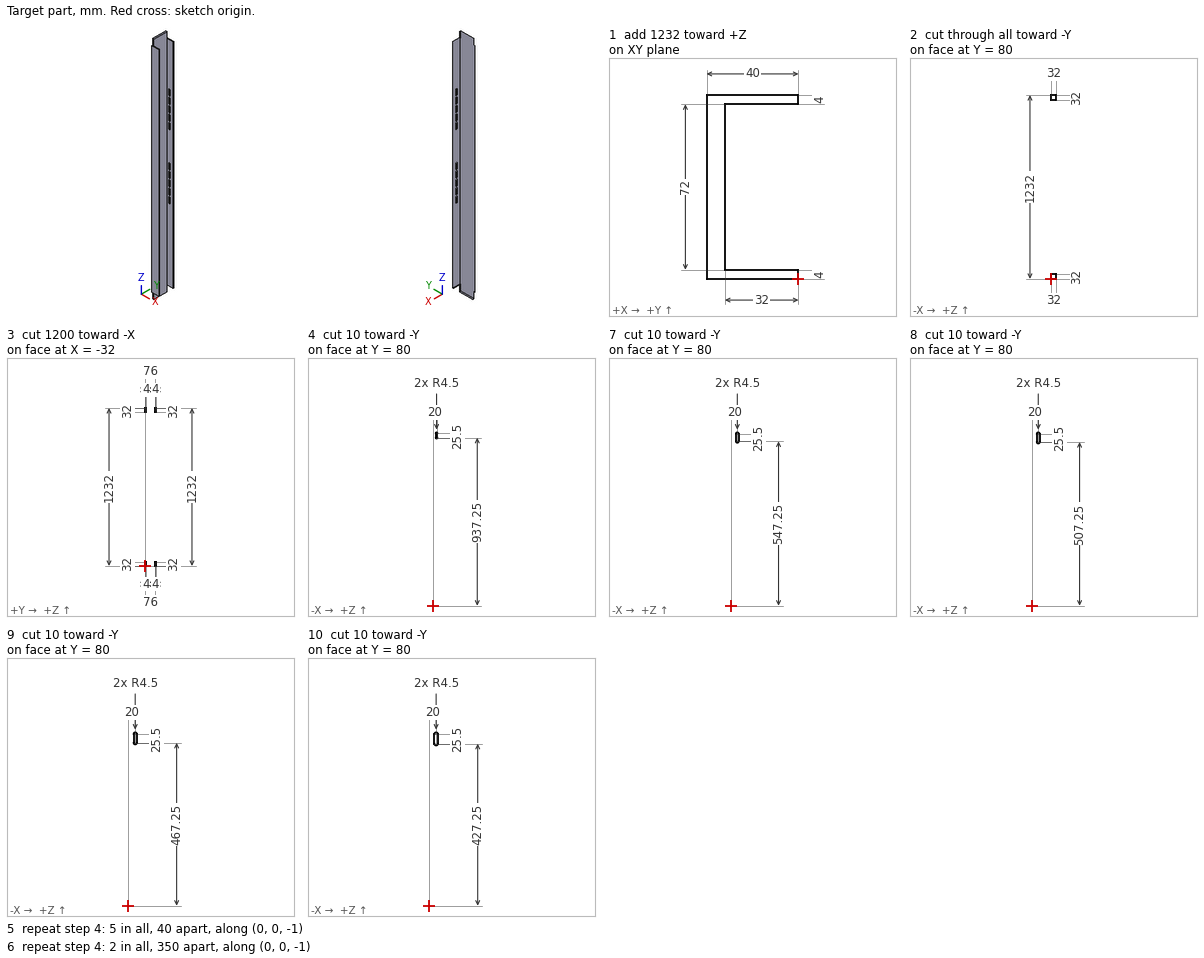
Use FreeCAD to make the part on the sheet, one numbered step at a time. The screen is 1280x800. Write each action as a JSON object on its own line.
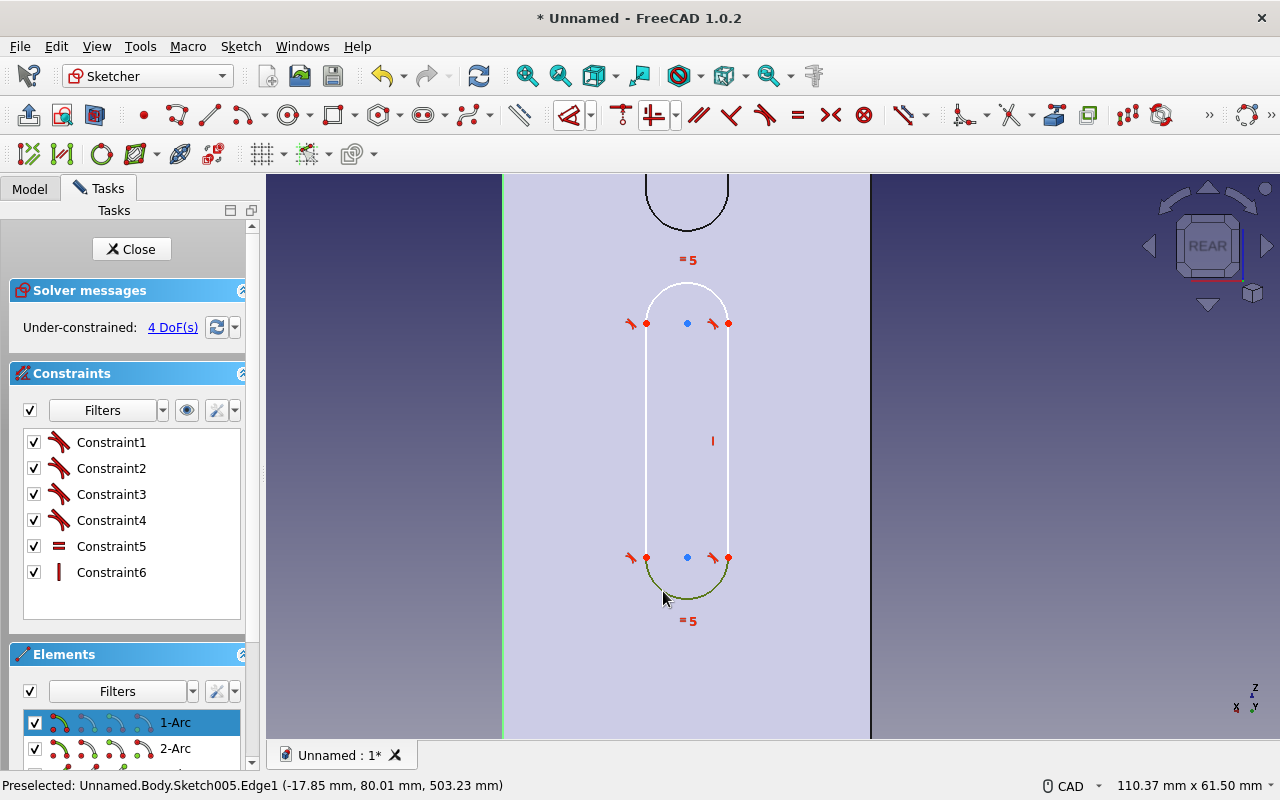
{"action": "key", "text": "k r"}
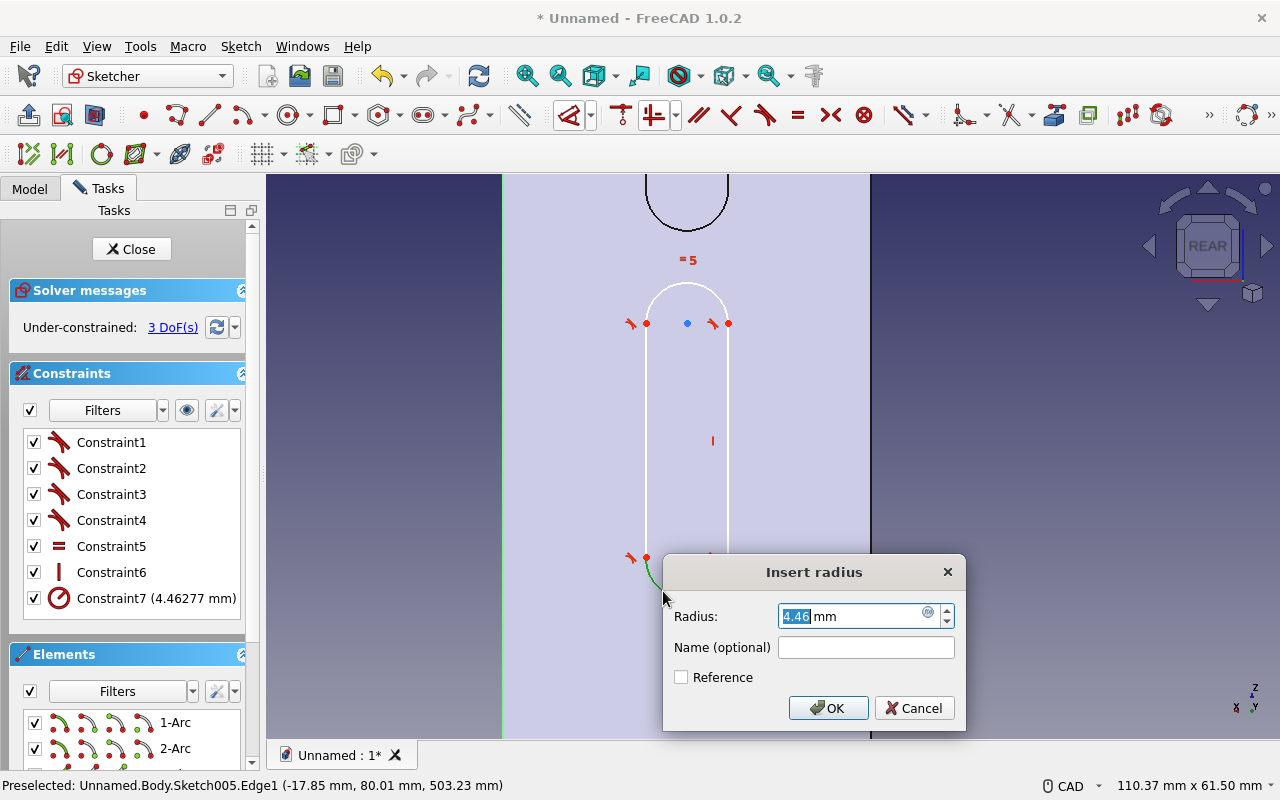
{"action": "type", "text": "4.5"}
{"action": "key", "text": "Return"}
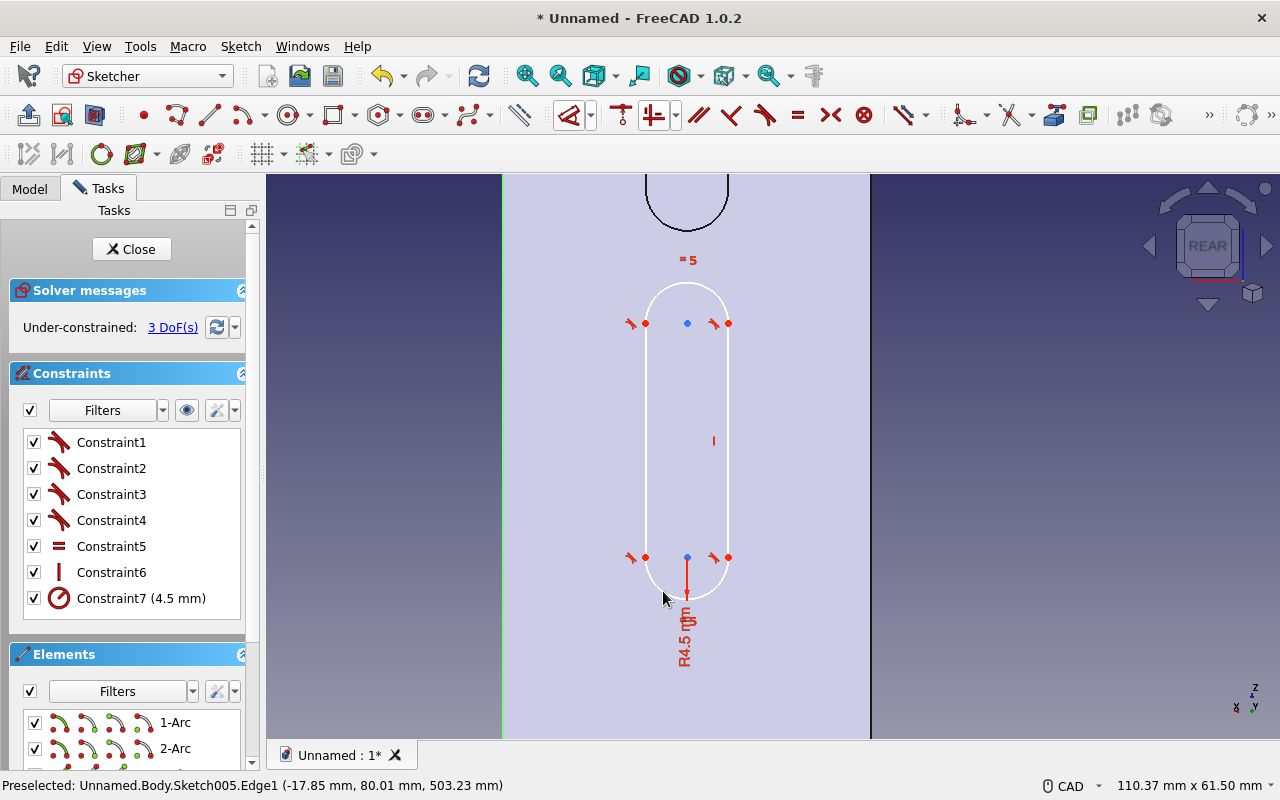
{"action": "left_click", "coordinate": [687, 558]}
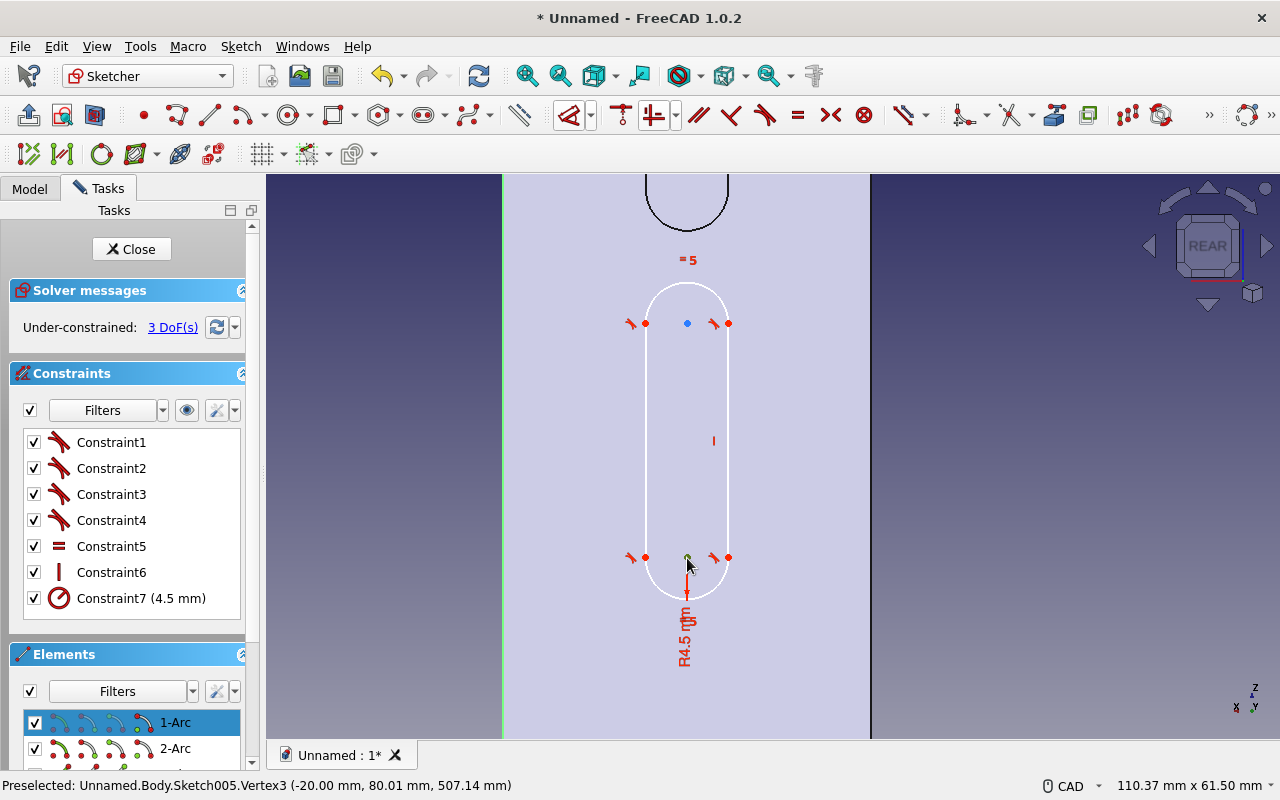
{"action": "left_click", "coordinate": [590, 116]}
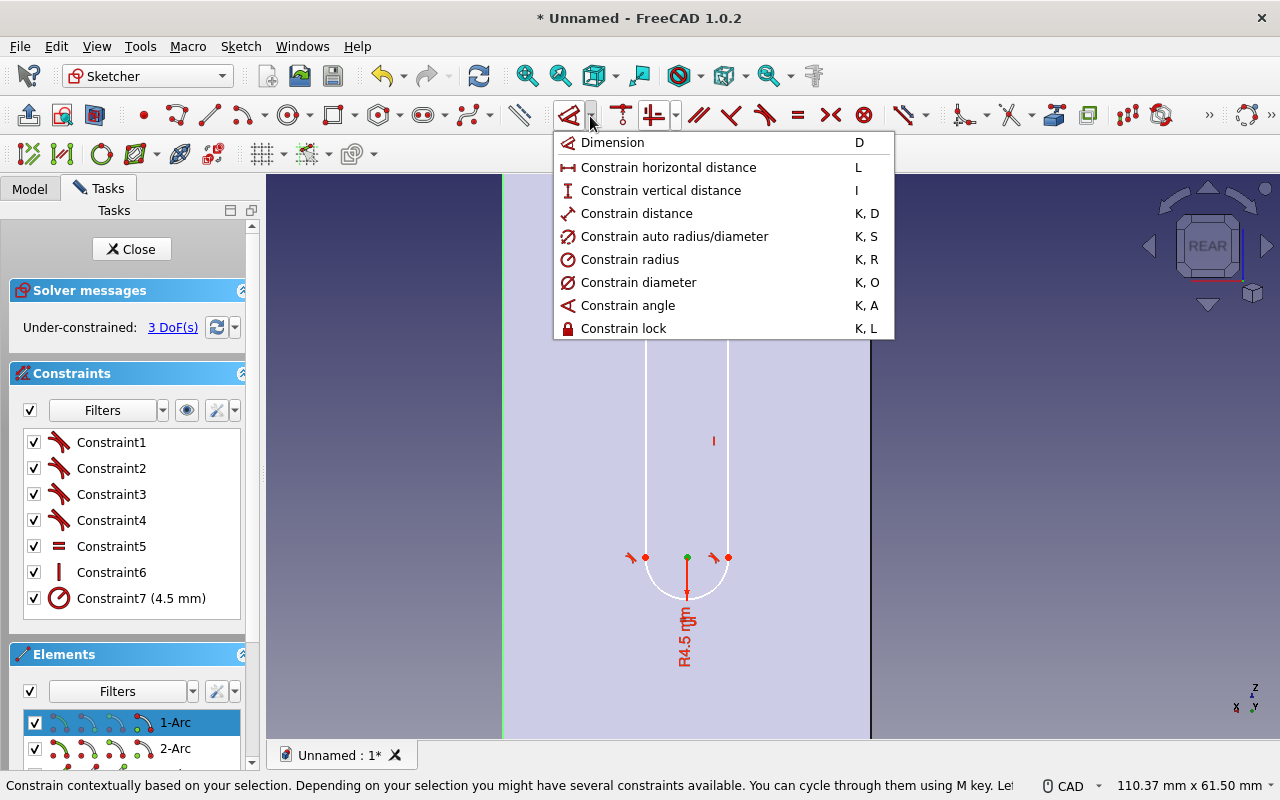
{"action": "left_click", "coordinate": [724, 168]}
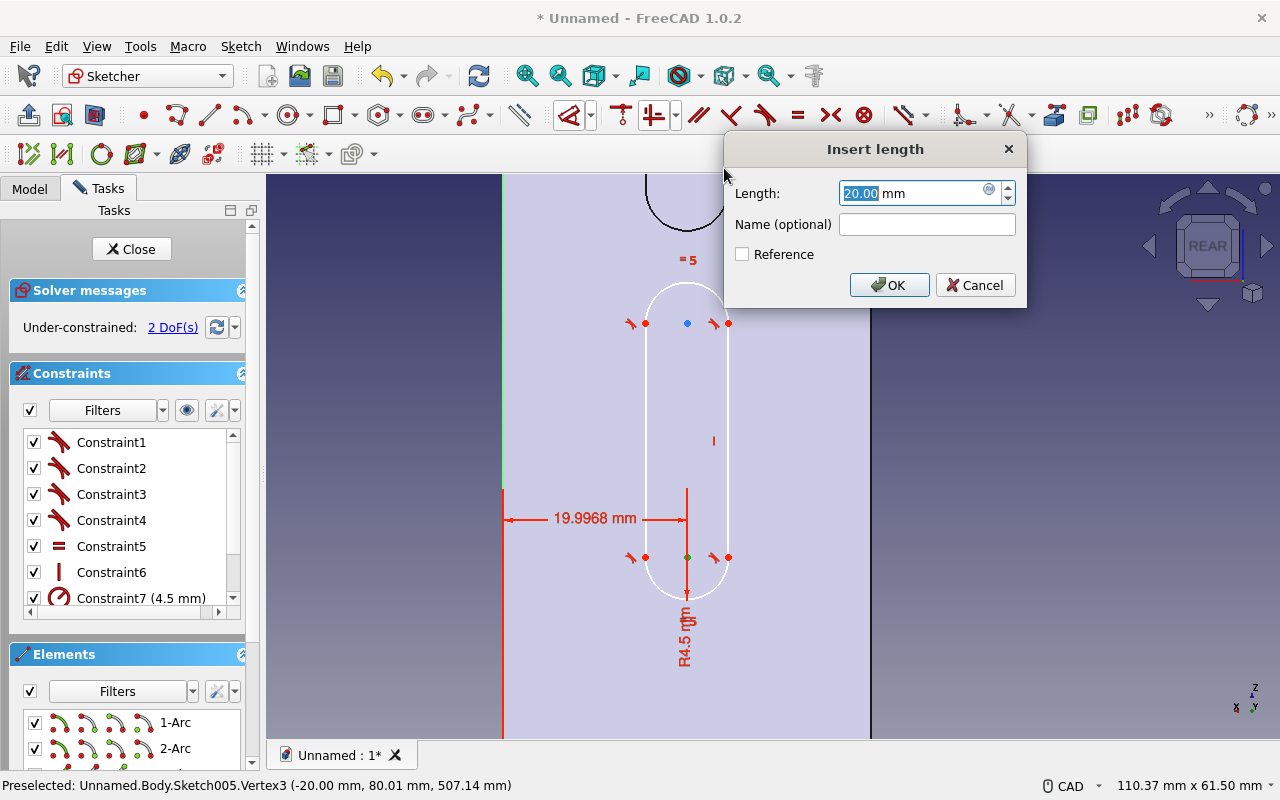
{"action": "type", "text": "20"}
{"action": "key", "text": "Return"}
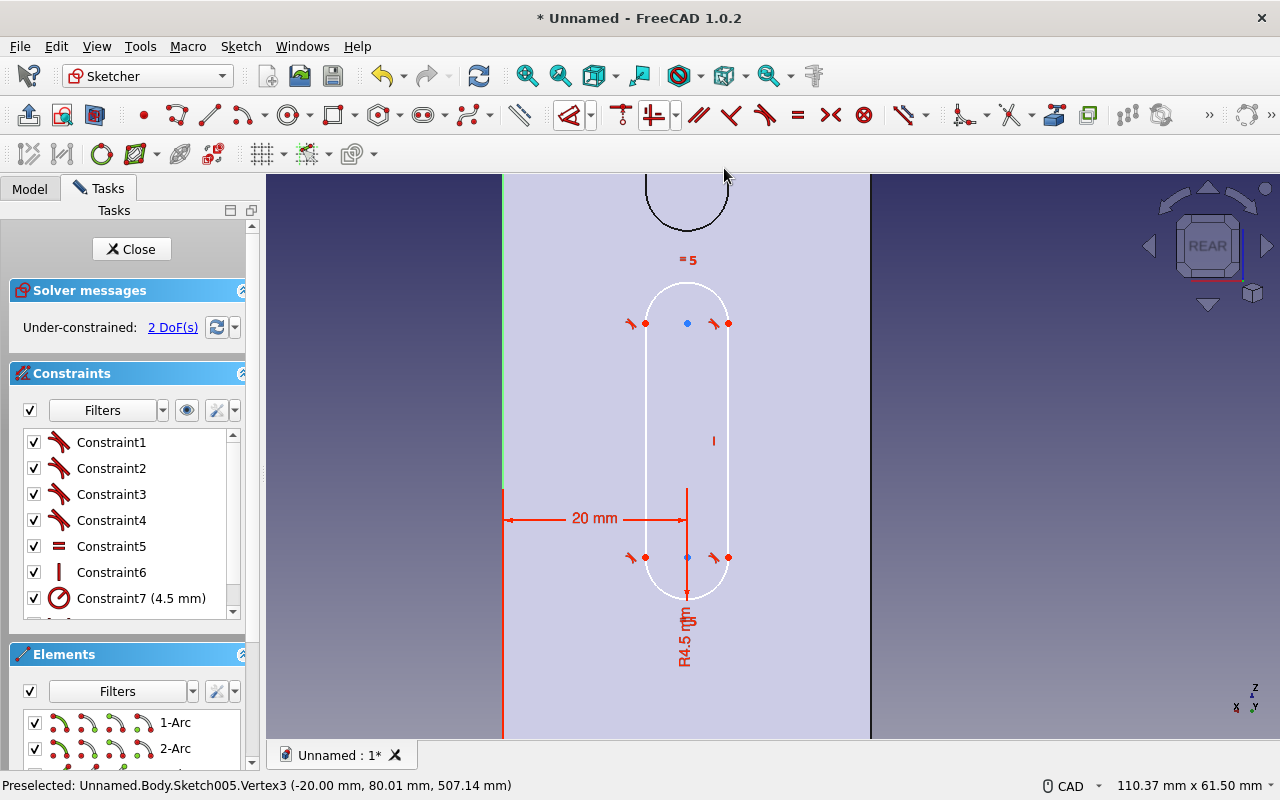
{"action": "left_click", "coordinate": [646, 488]}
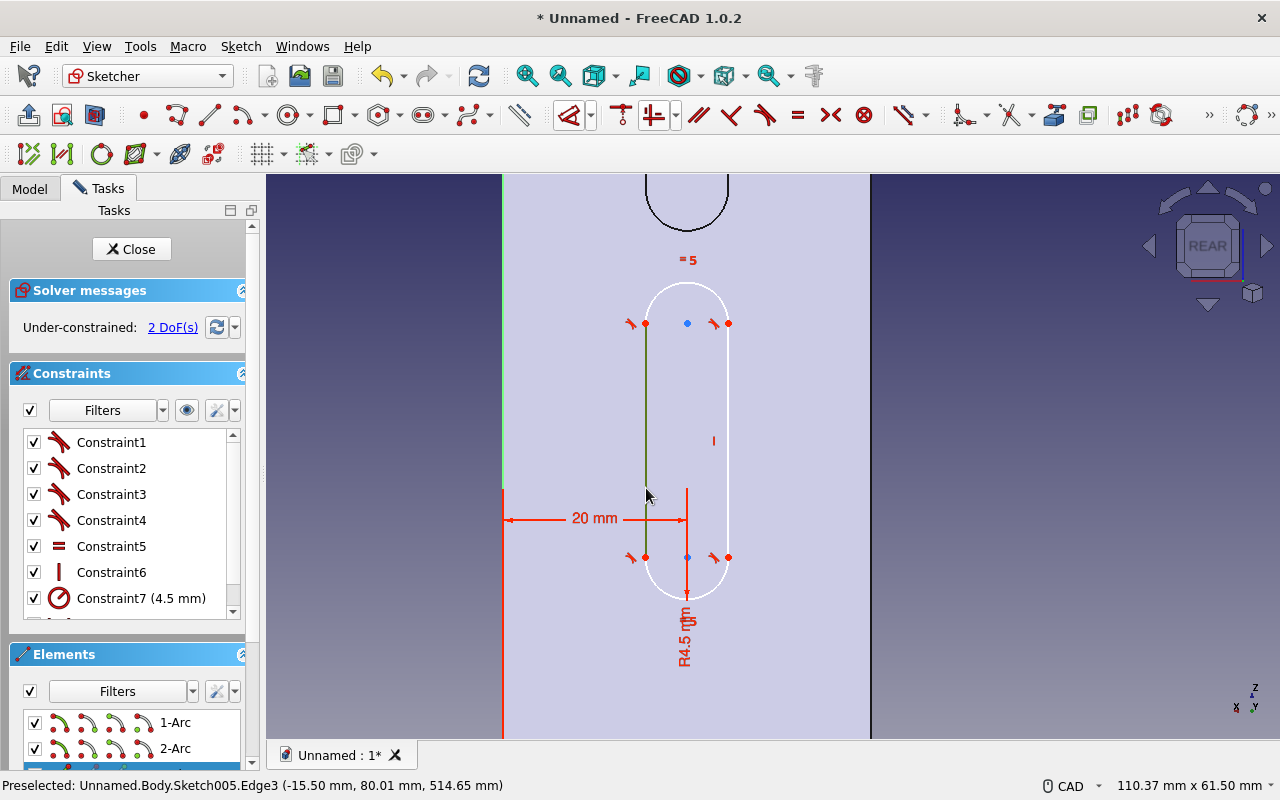
{"action": "left_click", "coordinate": [590, 116]}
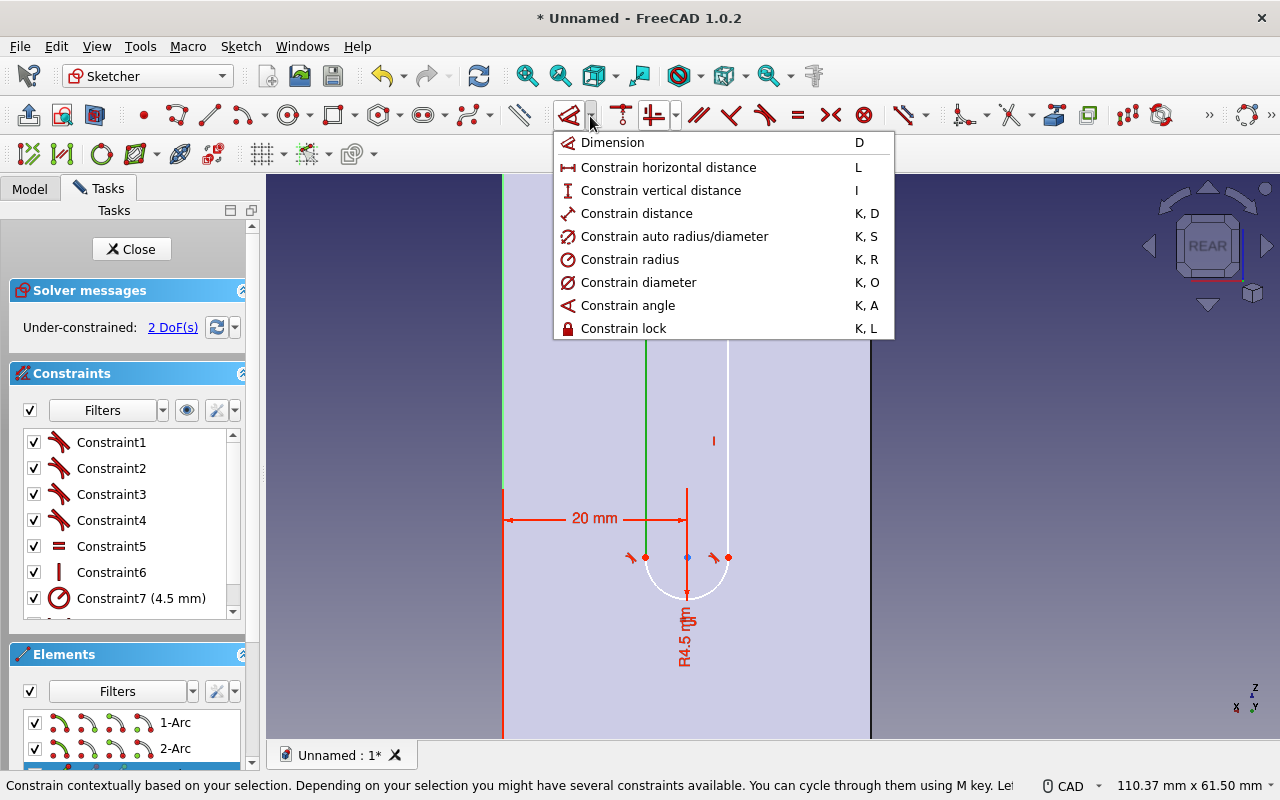
{"action": "left_click", "coordinate": [724, 190]}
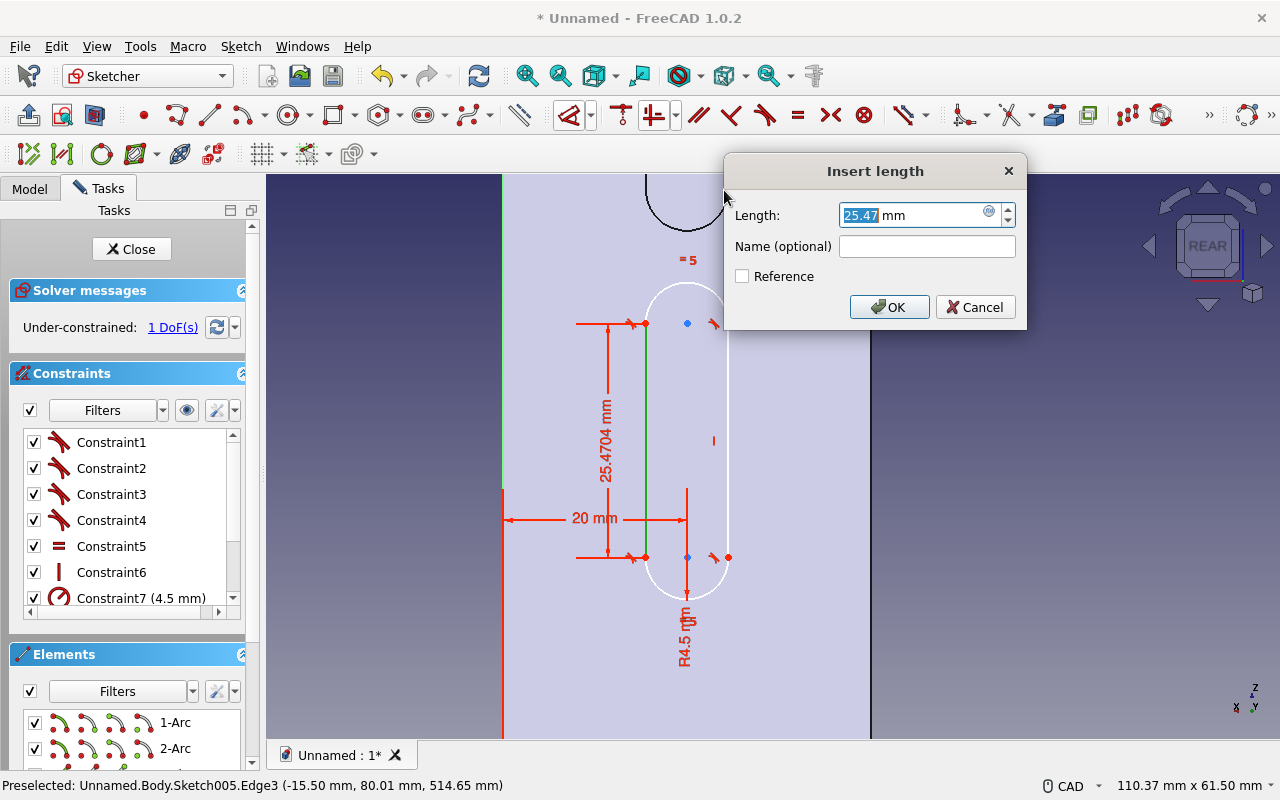
{"action": "type", "text": "25.5"}
{"action": "key", "text": "Return"}